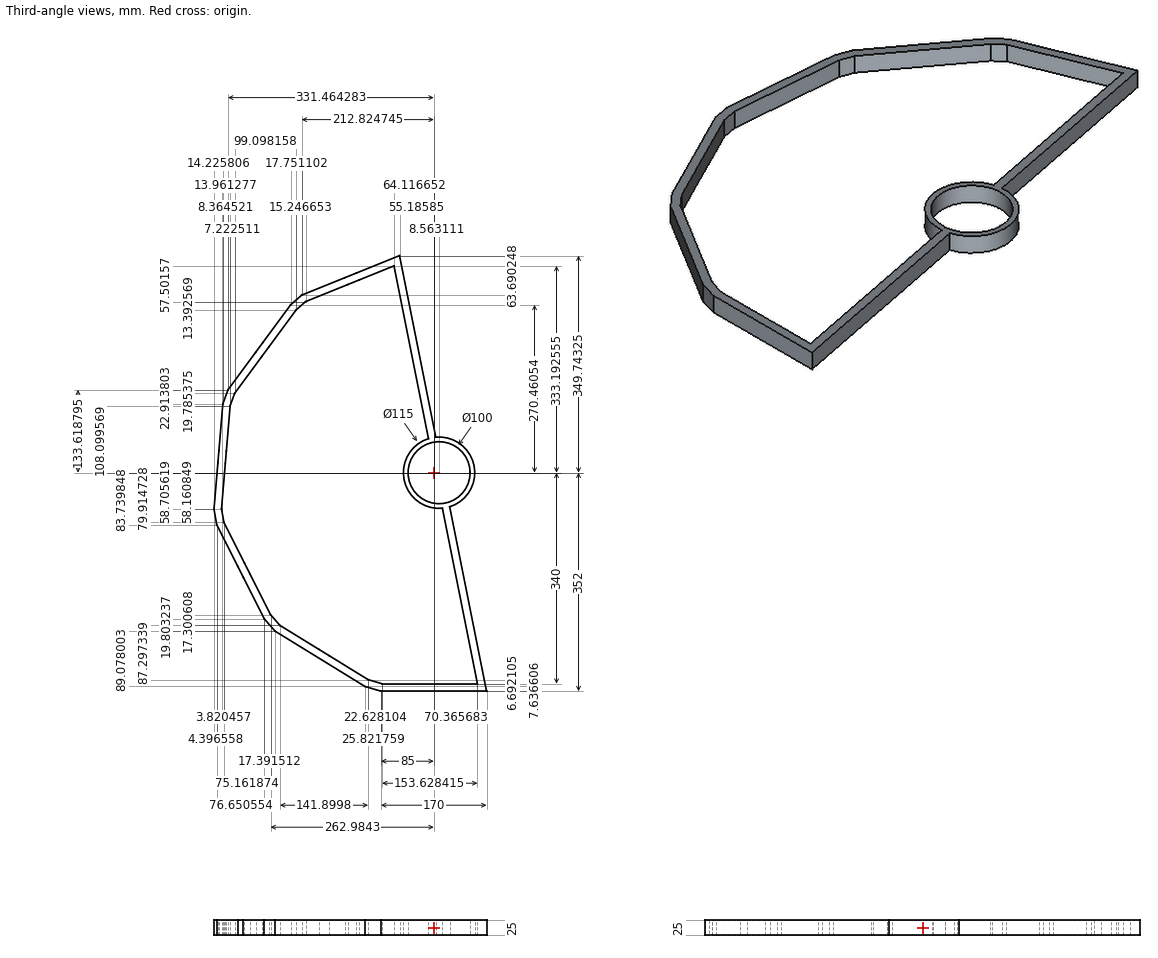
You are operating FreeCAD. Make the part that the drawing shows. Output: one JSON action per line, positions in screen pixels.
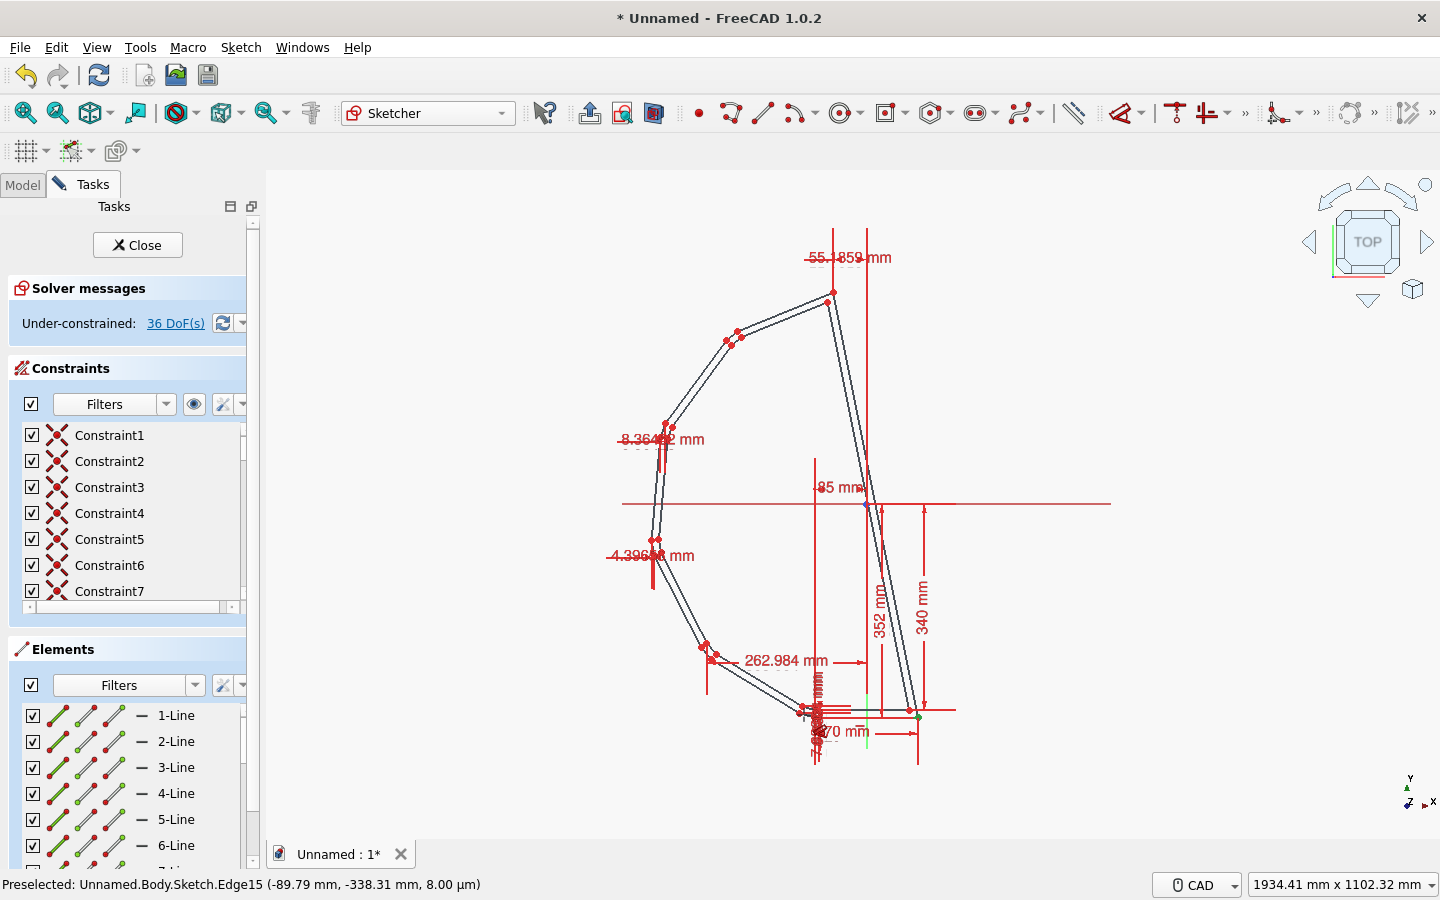
{"action": "scroll", "coordinate": [776, 691], "scroll_direction": "up", "scroll_amount": 4}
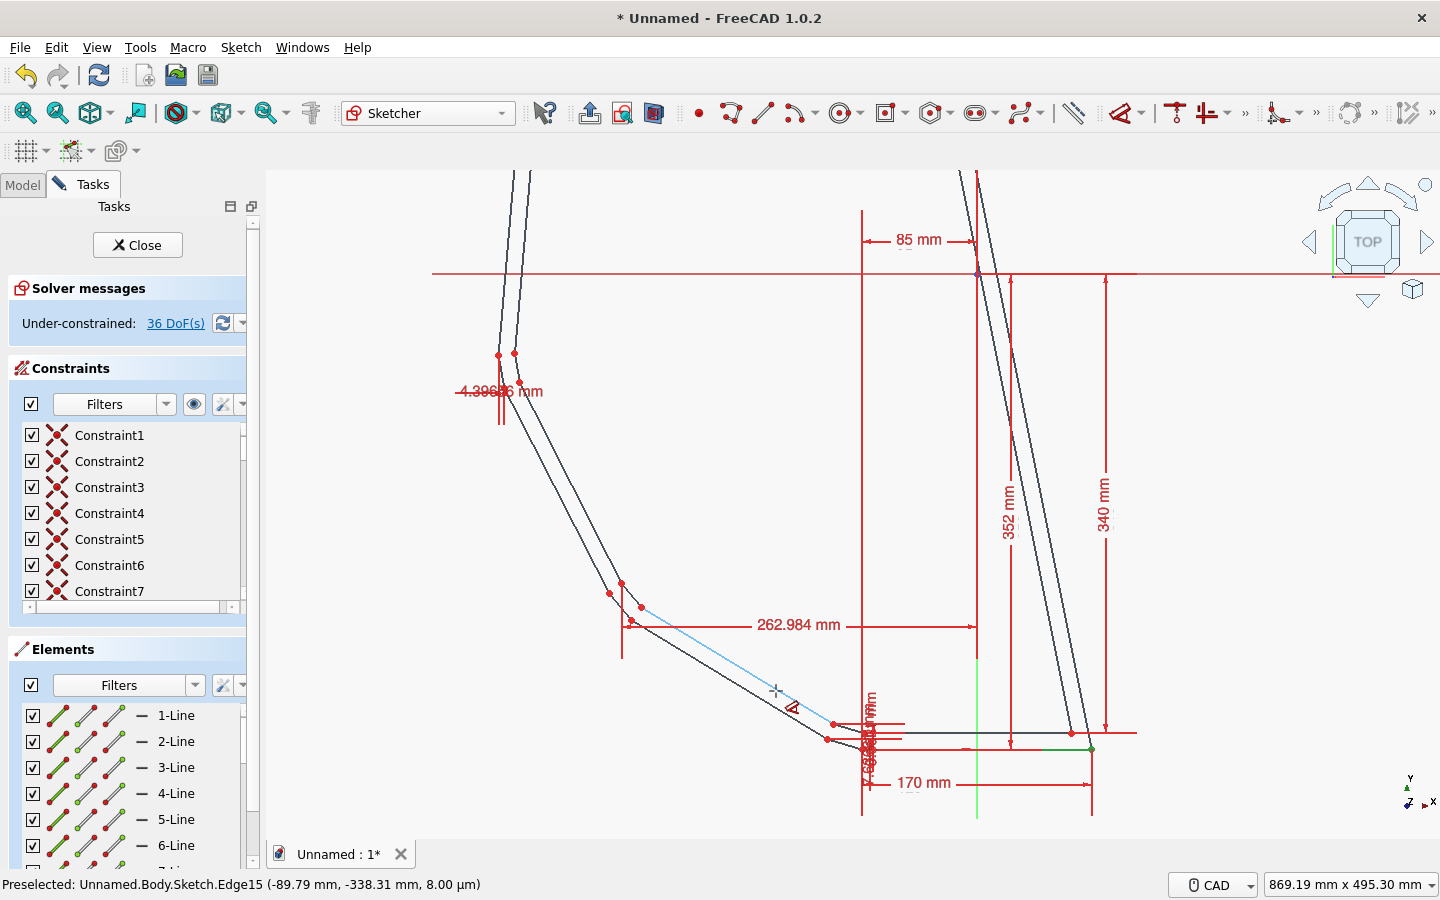
{"action": "left_click", "coordinate": [776, 689]}
{"action": "left_click", "coordinate": [738, 758]}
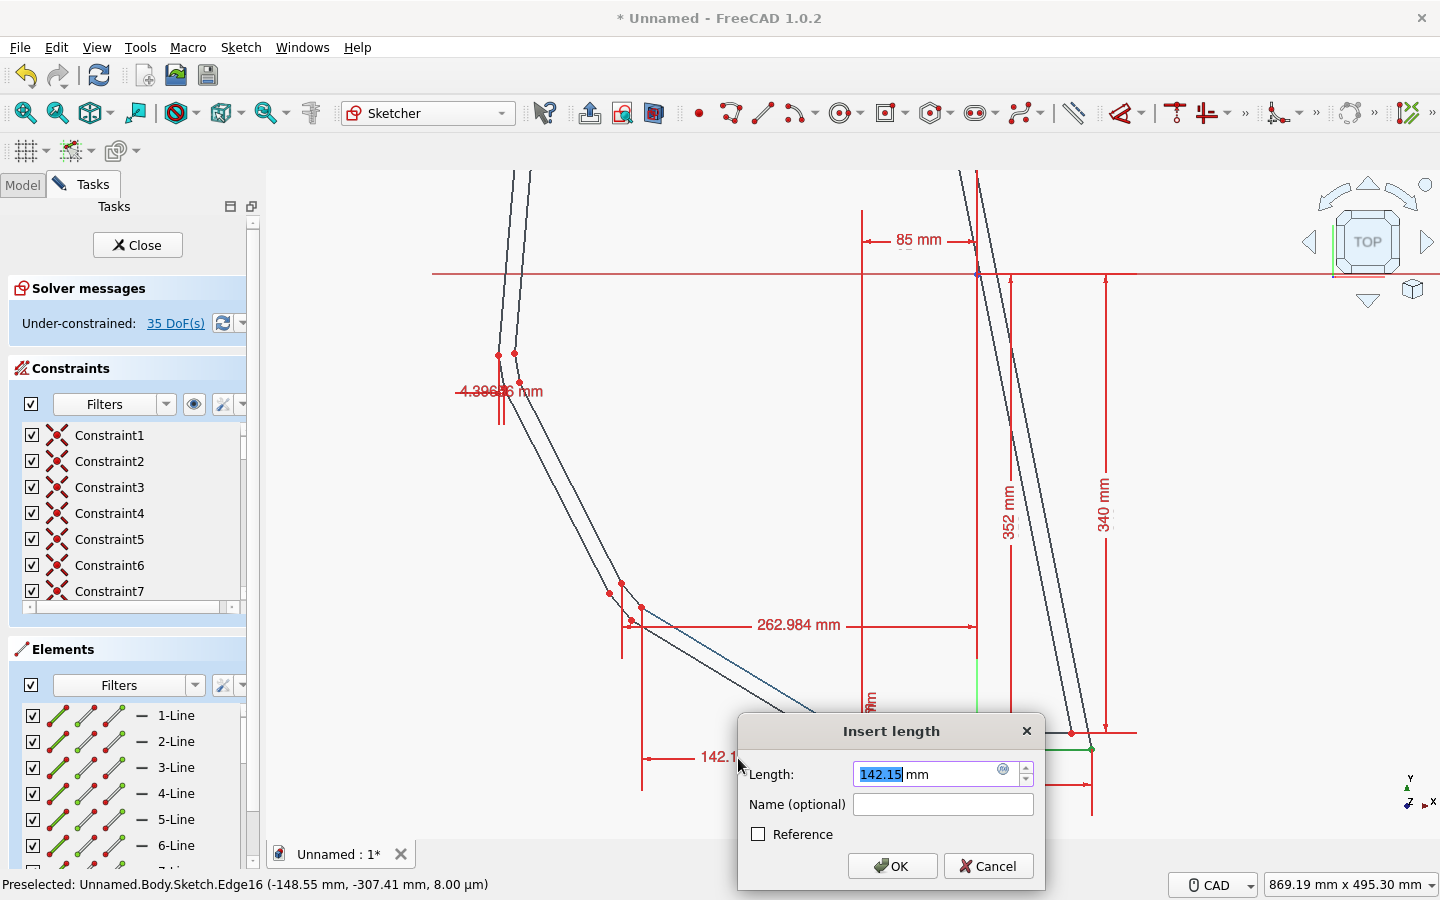
{"action": "type", "text": "141.8998"}
{"action": "key", "text": "Return"}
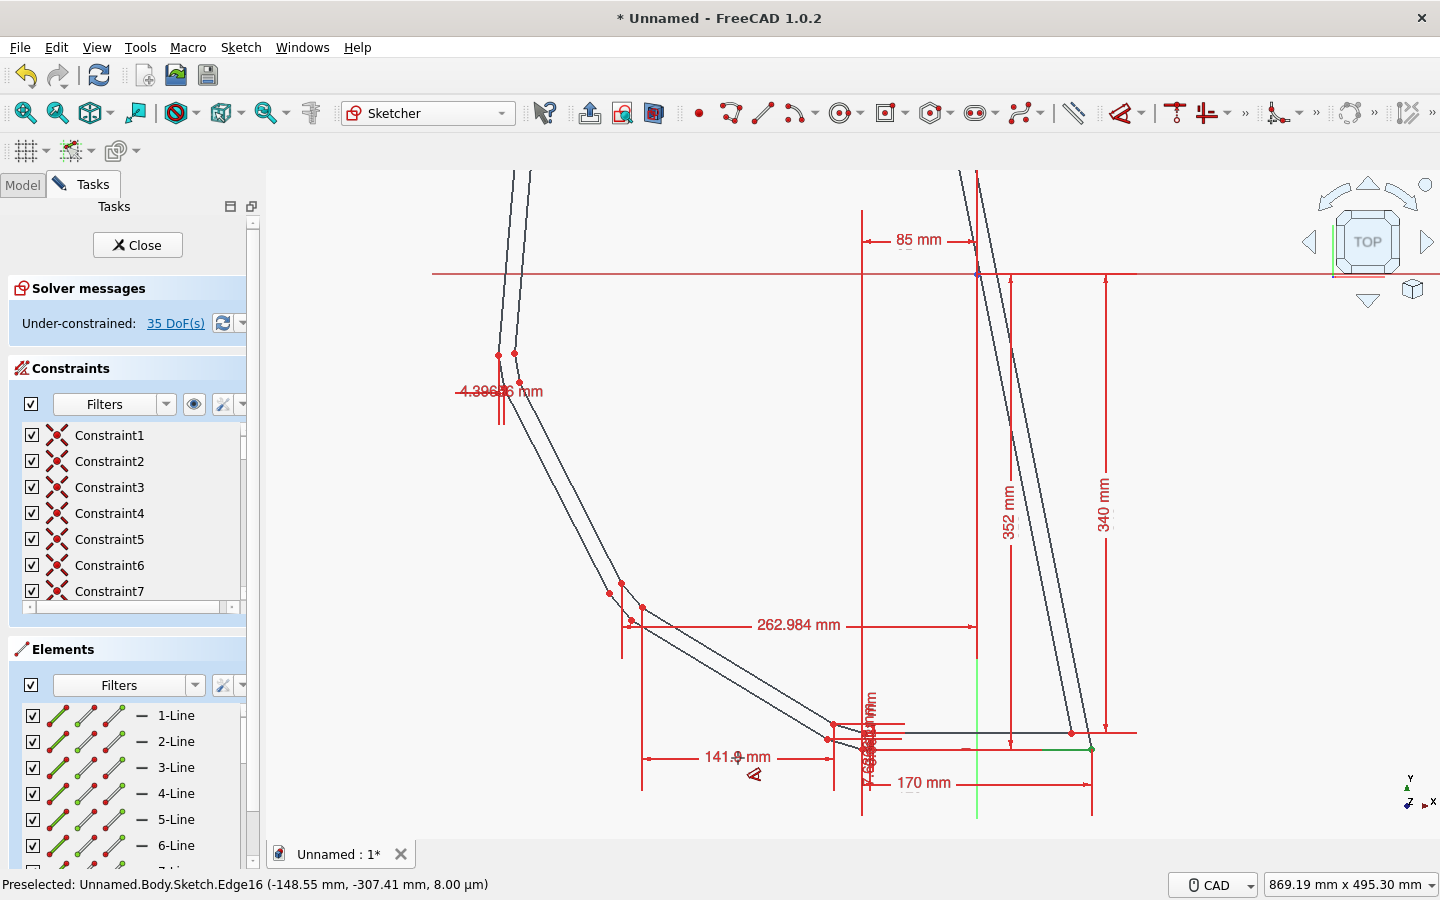
{"action": "scroll", "coordinate": [518, 371], "scroll_direction": "up", "scroll_amount": 11}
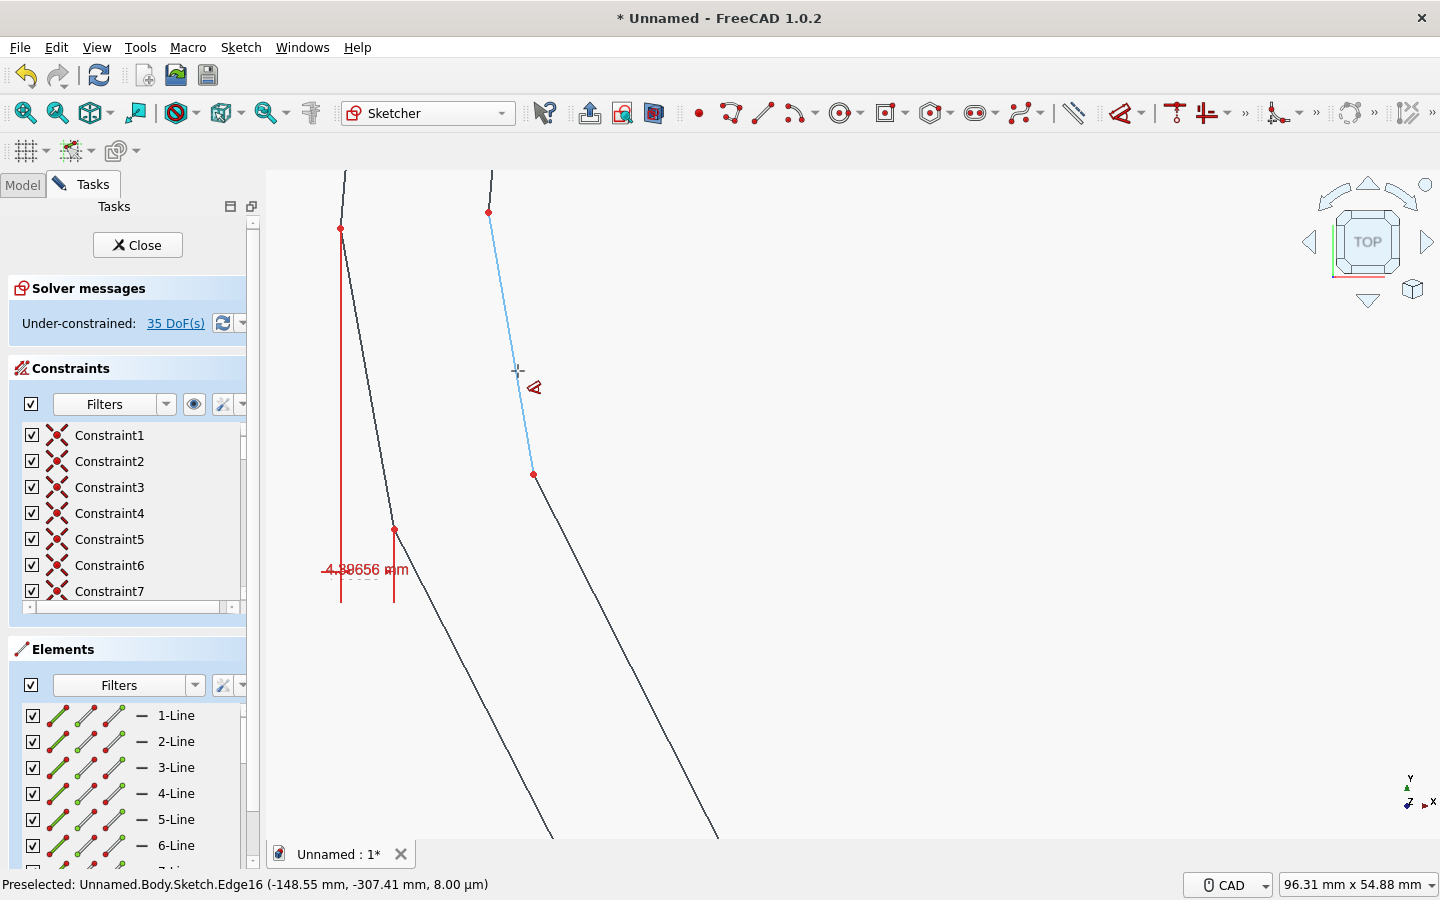
{"action": "left_click", "coordinate": [516, 370]}
{"action": "left_click", "coordinate": [511, 509]}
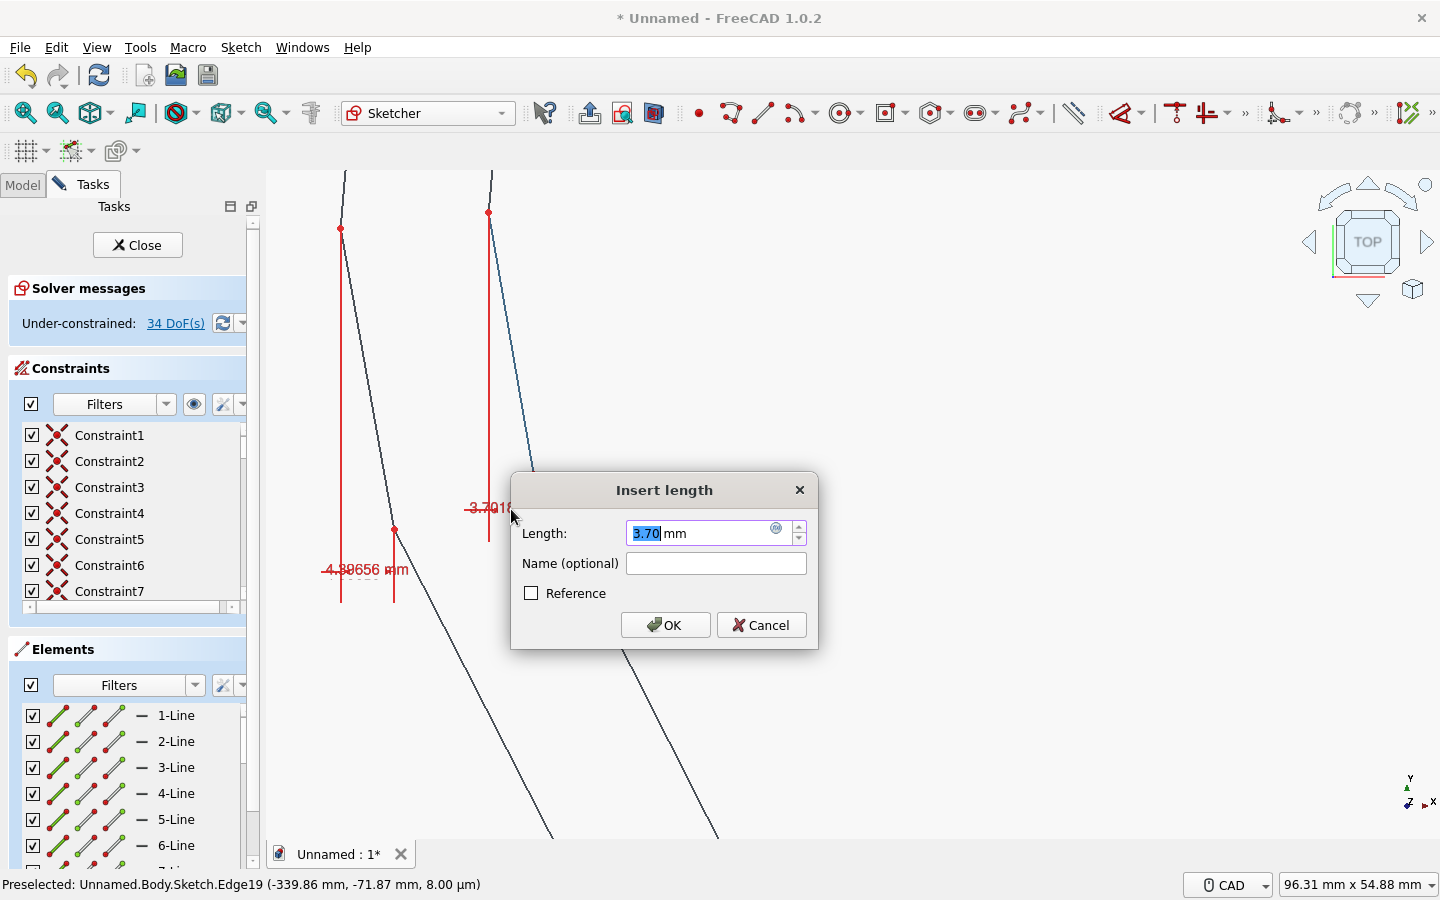
{"action": "type", "text": "3.820457"}
{"action": "key", "text": "Return"}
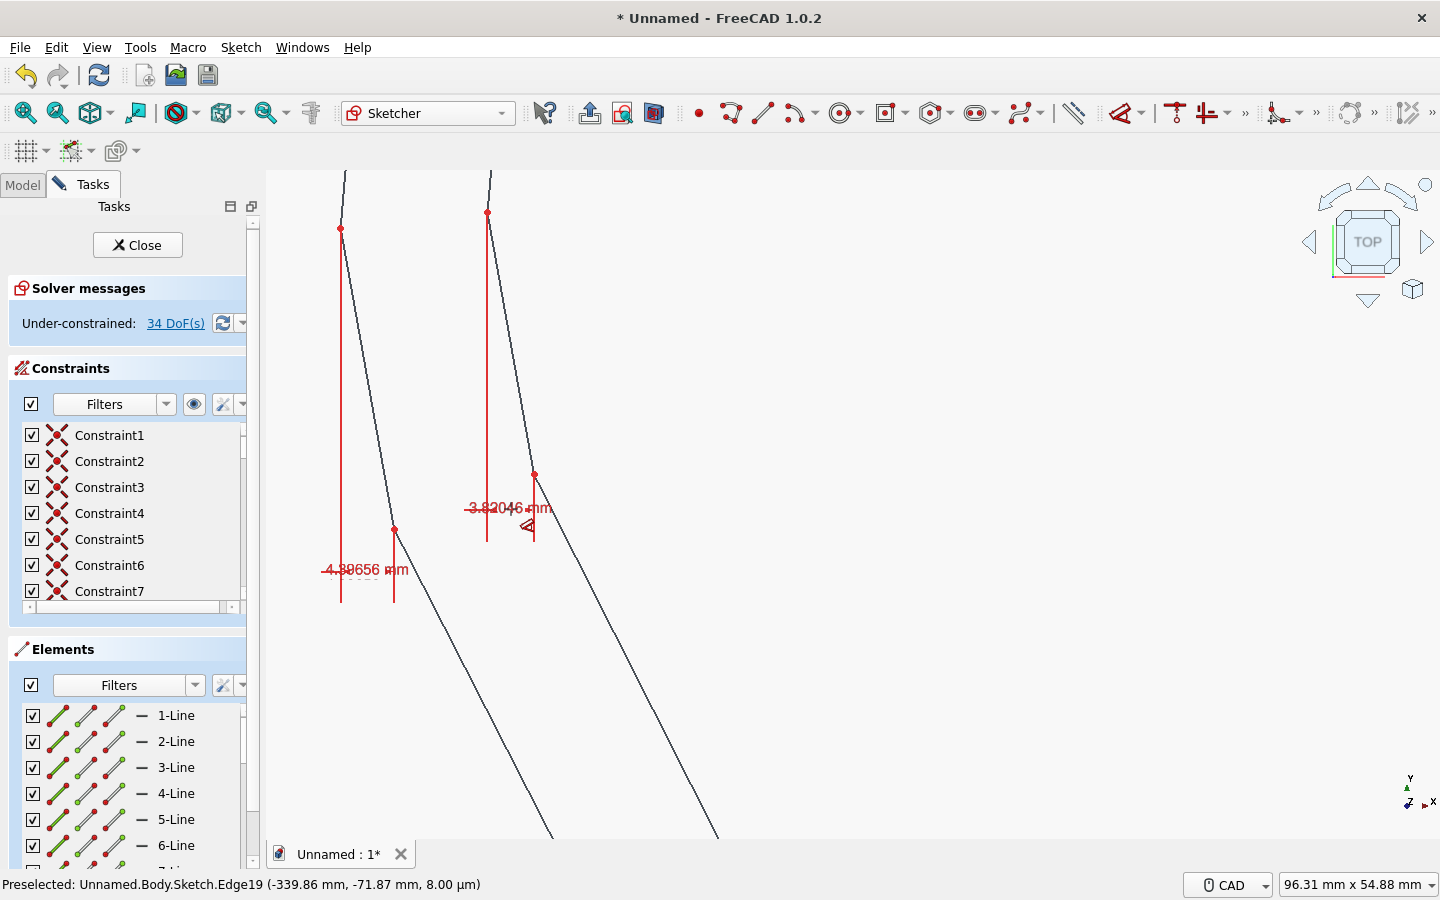
{"action": "scroll", "coordinate": [667, 557], "scroll_direction": "down", "scroll_amount": 15}